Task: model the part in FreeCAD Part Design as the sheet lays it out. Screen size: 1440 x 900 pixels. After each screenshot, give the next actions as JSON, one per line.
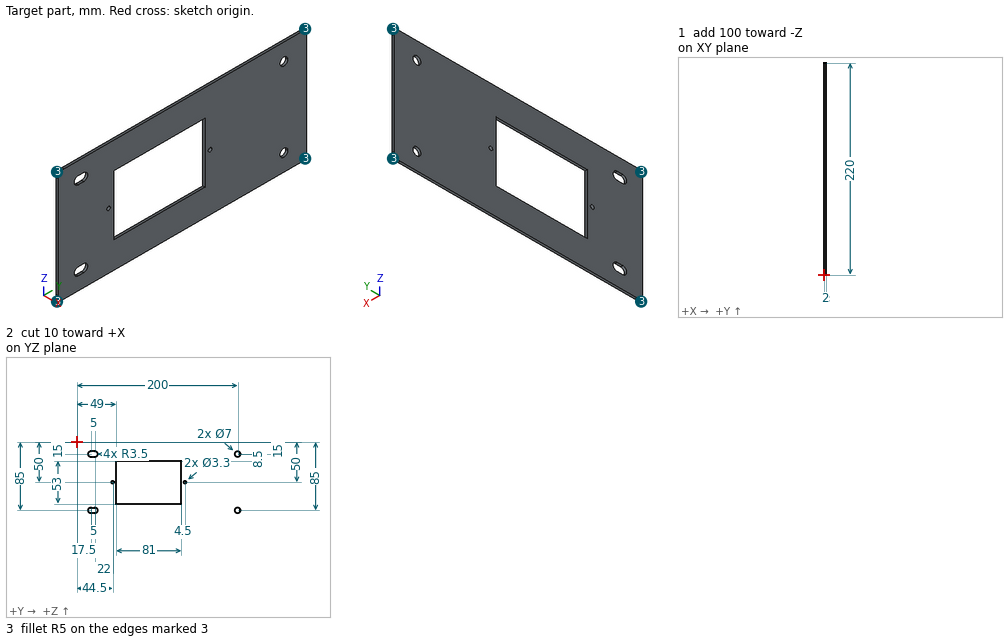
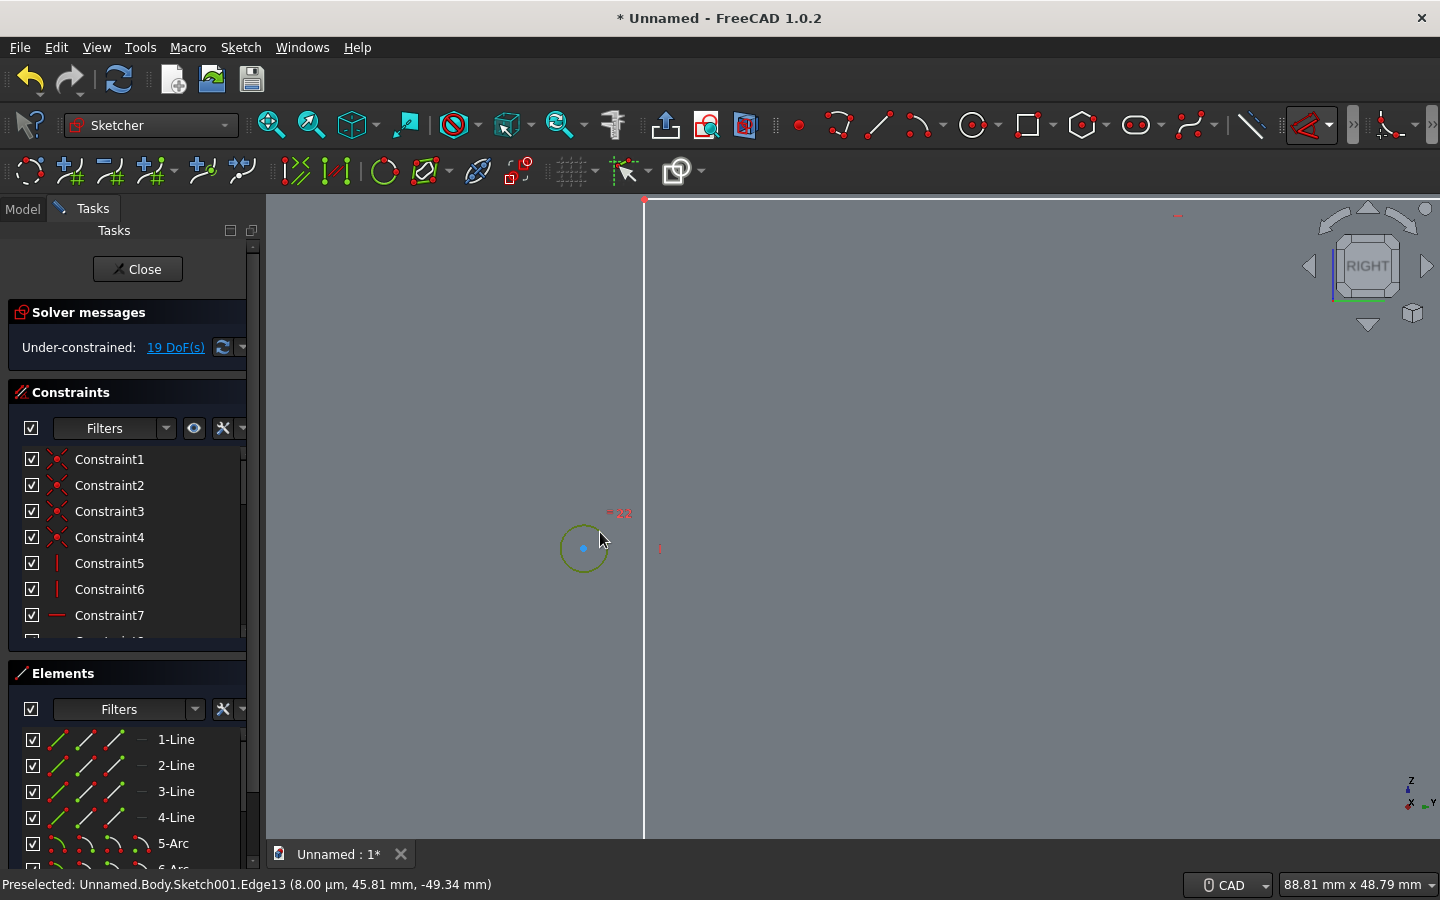
{"action": "key", "text": "k o"}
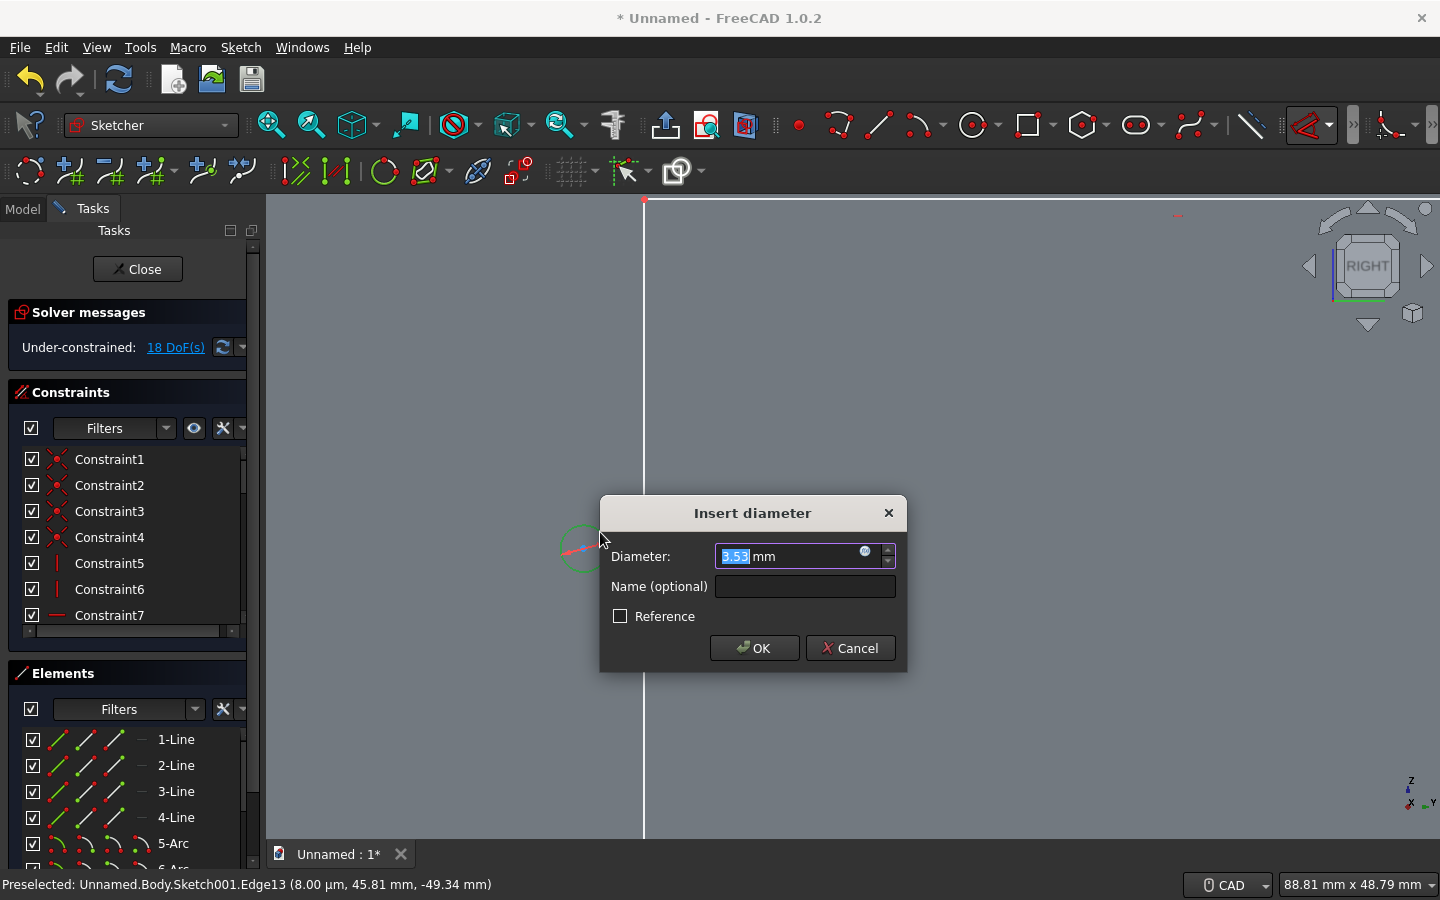
{"action": "type", "text": "3.3"}
{"action": "key", "text": "Return"}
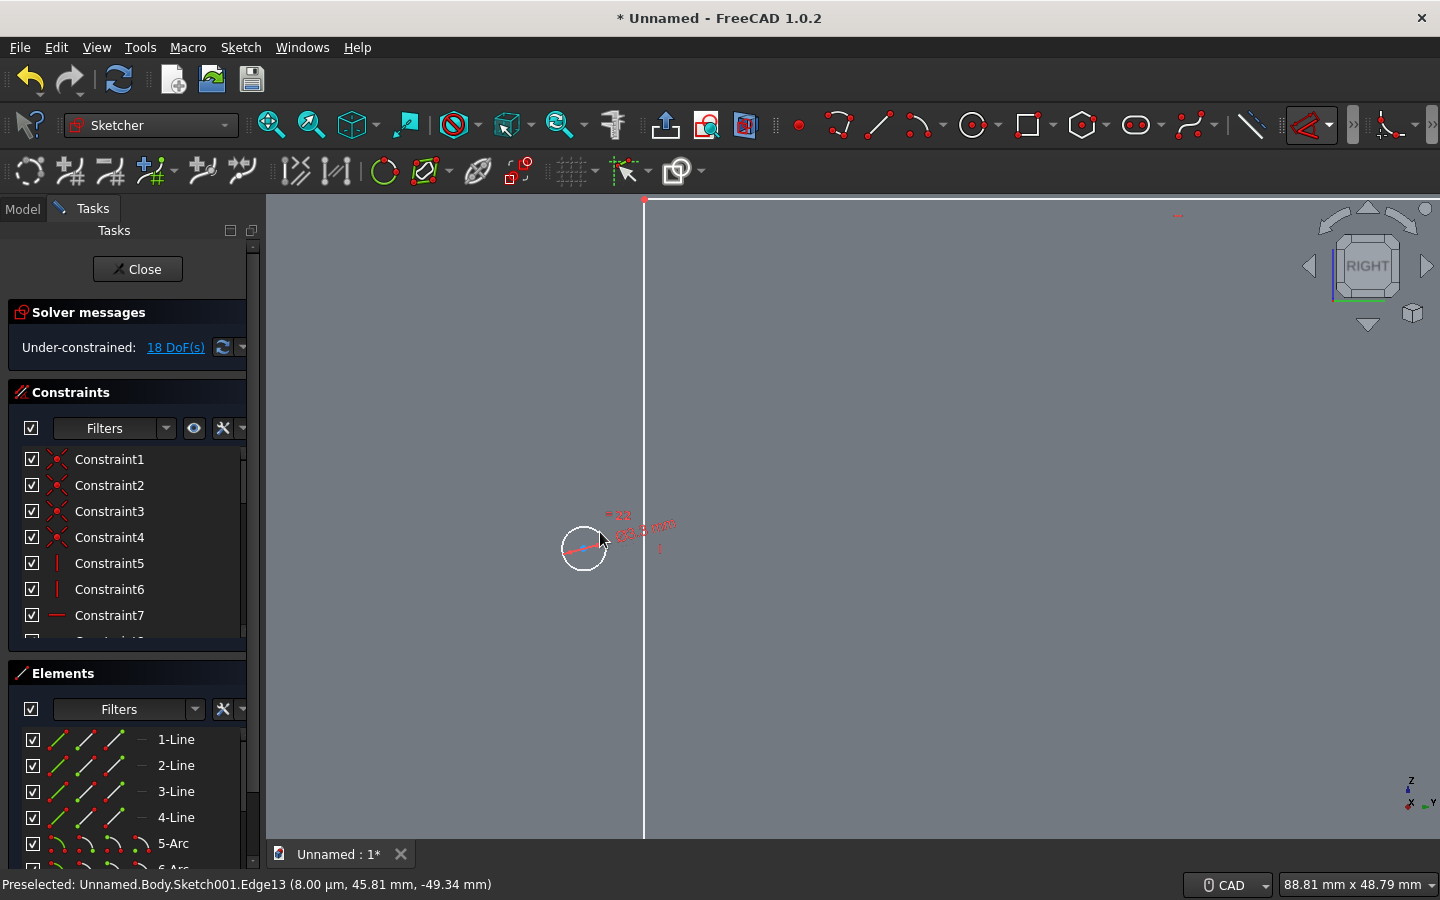
{"action": "scroll", "coordinate": [602, 532], "scroll_direction": "down", "scroll_amount": 7}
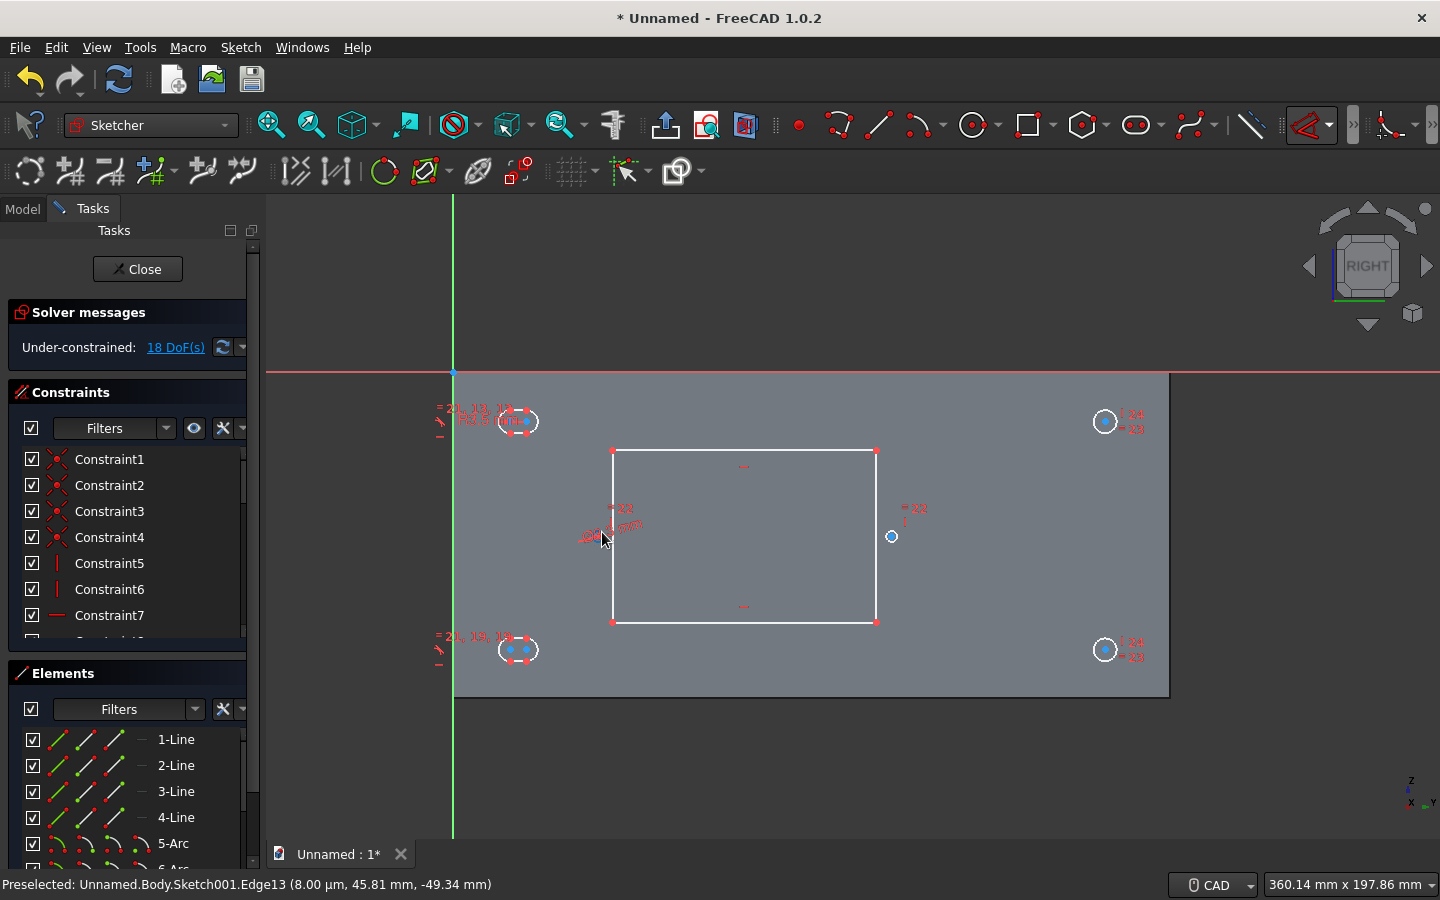
{"action": "scroll", "coordinate": [1113, 414], "scroll_direction": "up", "scroll_amount": 3}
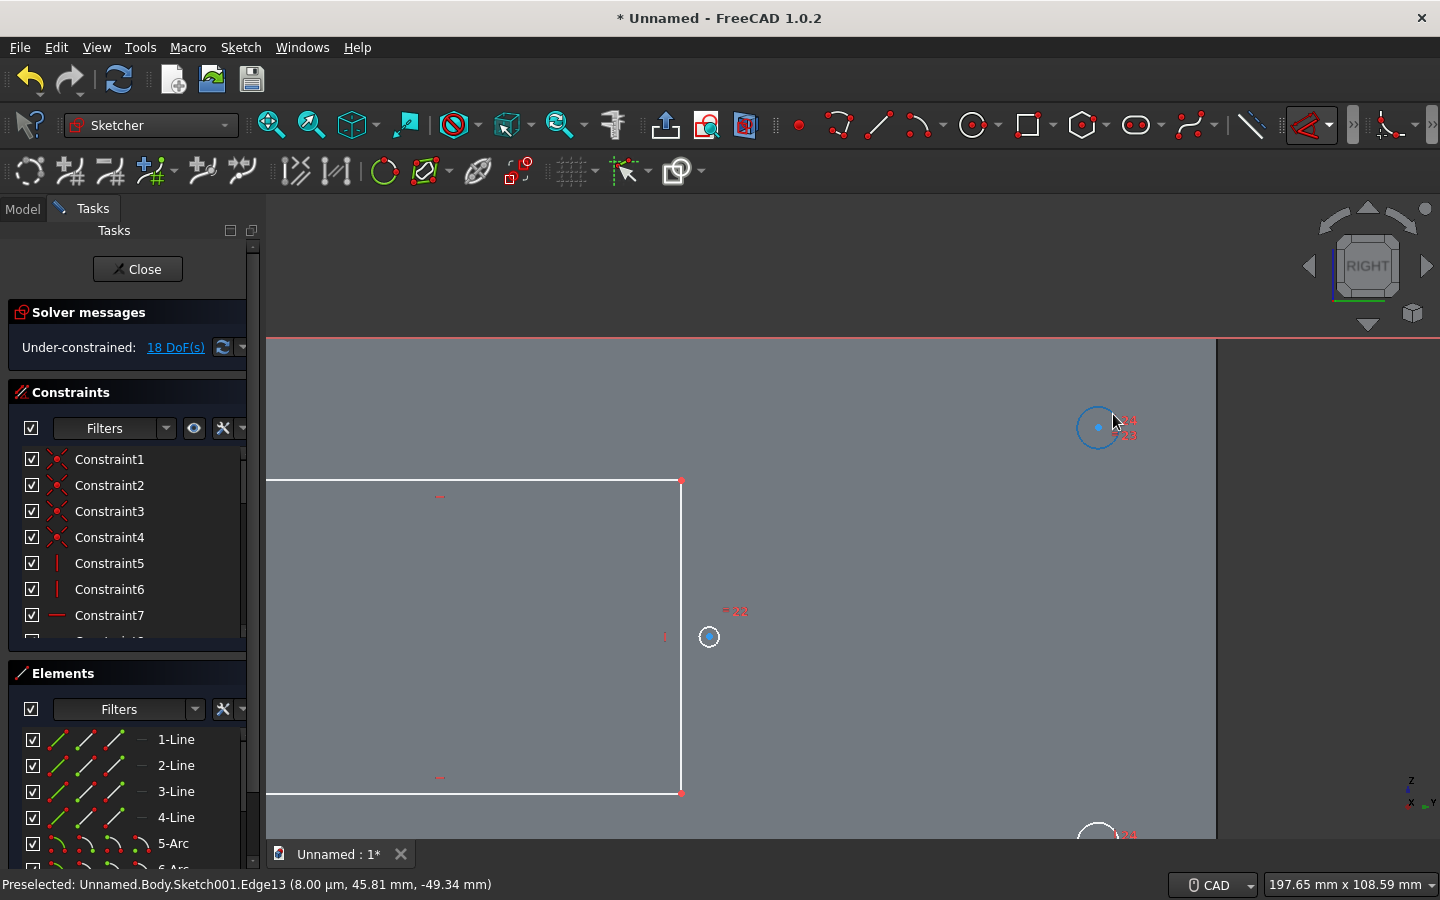
{"action": "left_click", "coordinate": [1083, 413]}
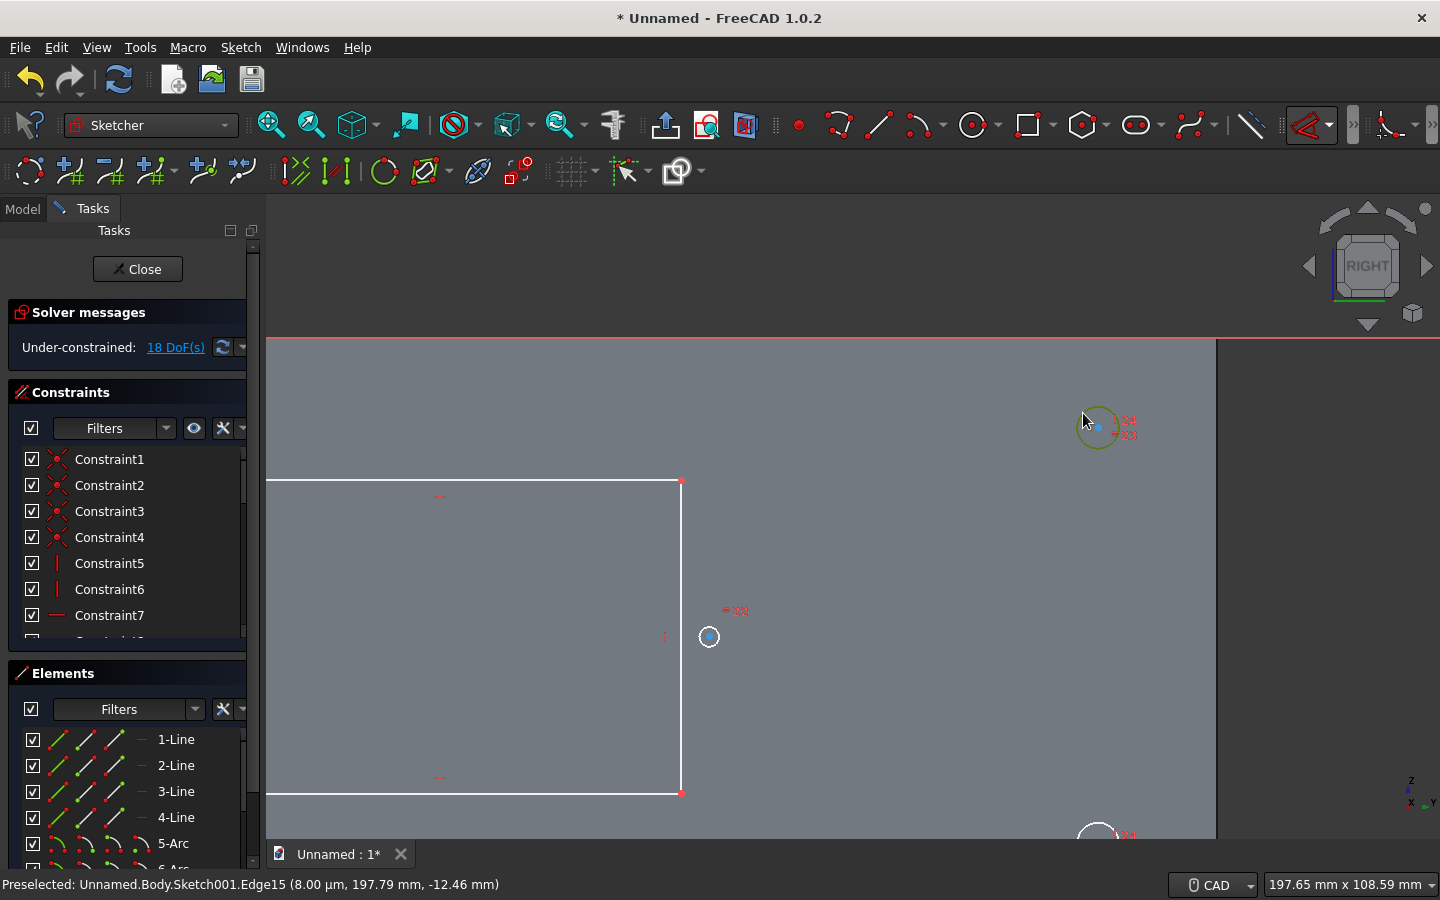
{"action": "key", "text": "k o"}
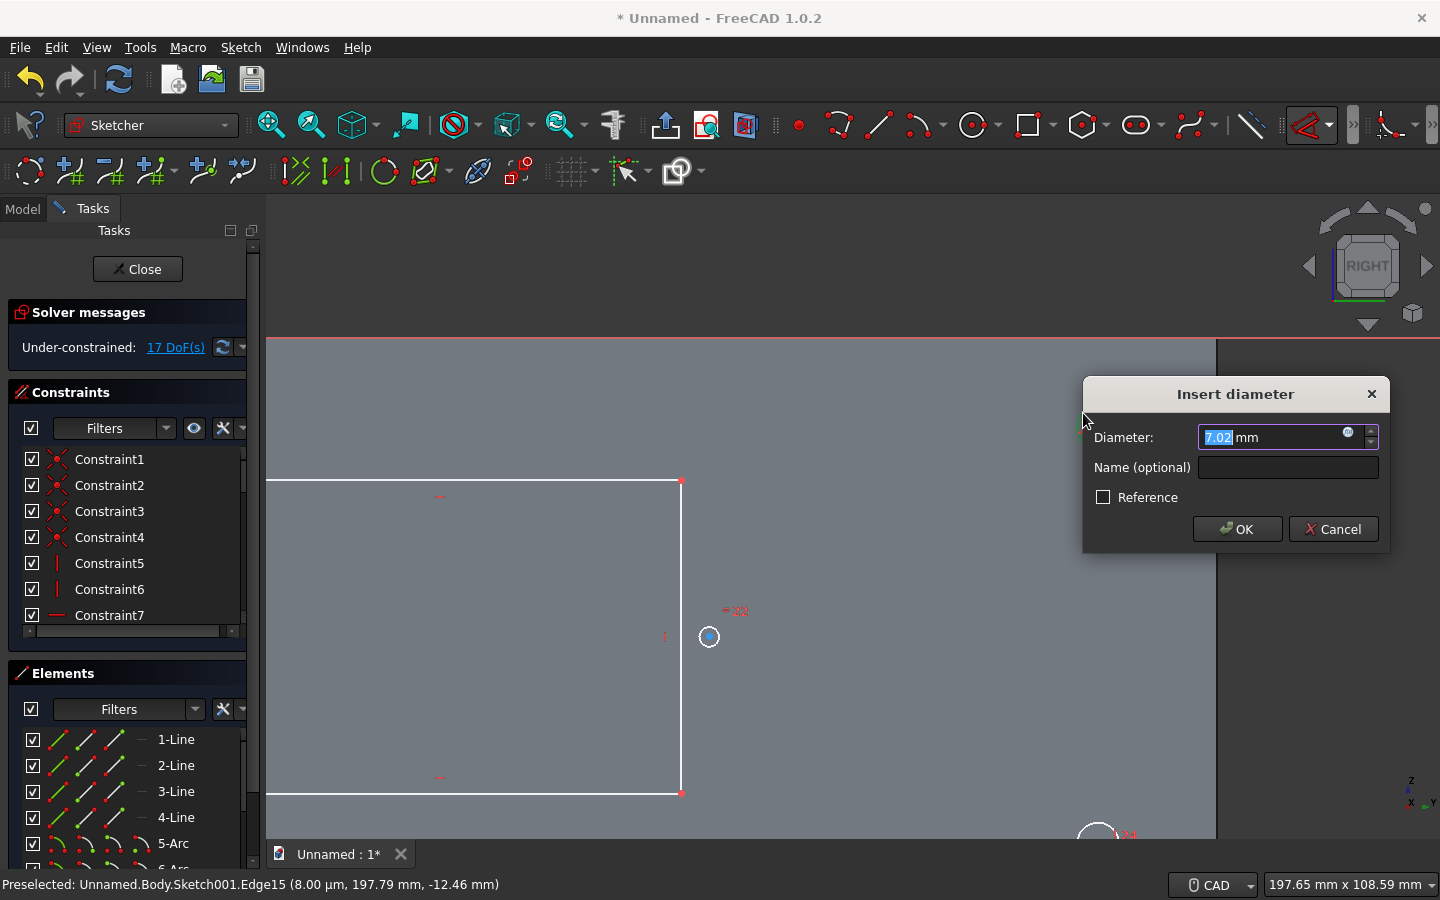
{"action": "type", "text": "7"}
{"action": "key", "text": "Return"}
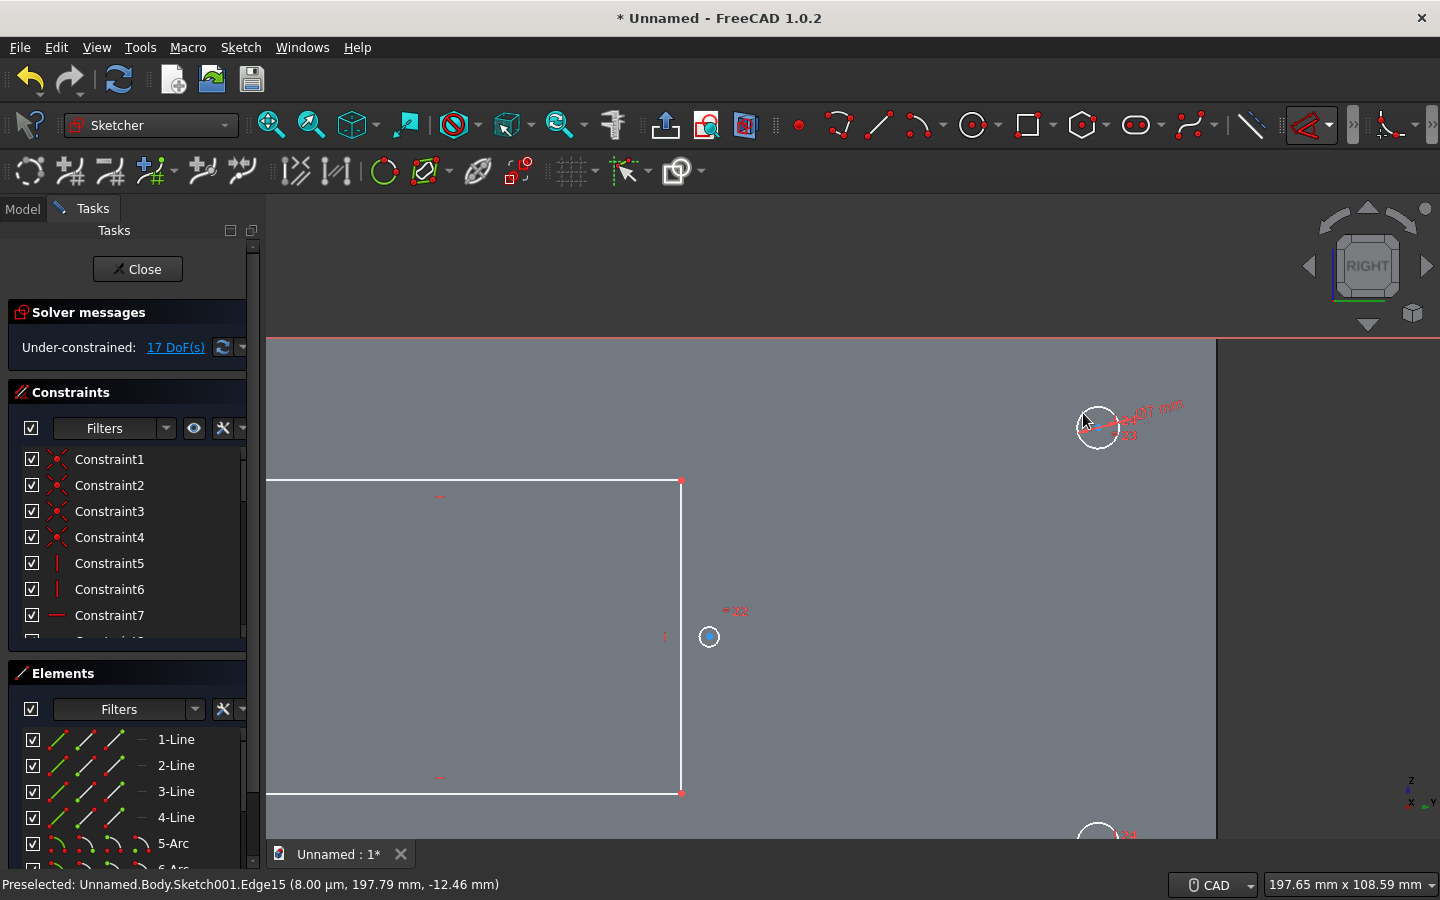
{"action": "scroll", "coordinate": [1113, 414], "scroll_direction": "down", "scroll_amount": 3}